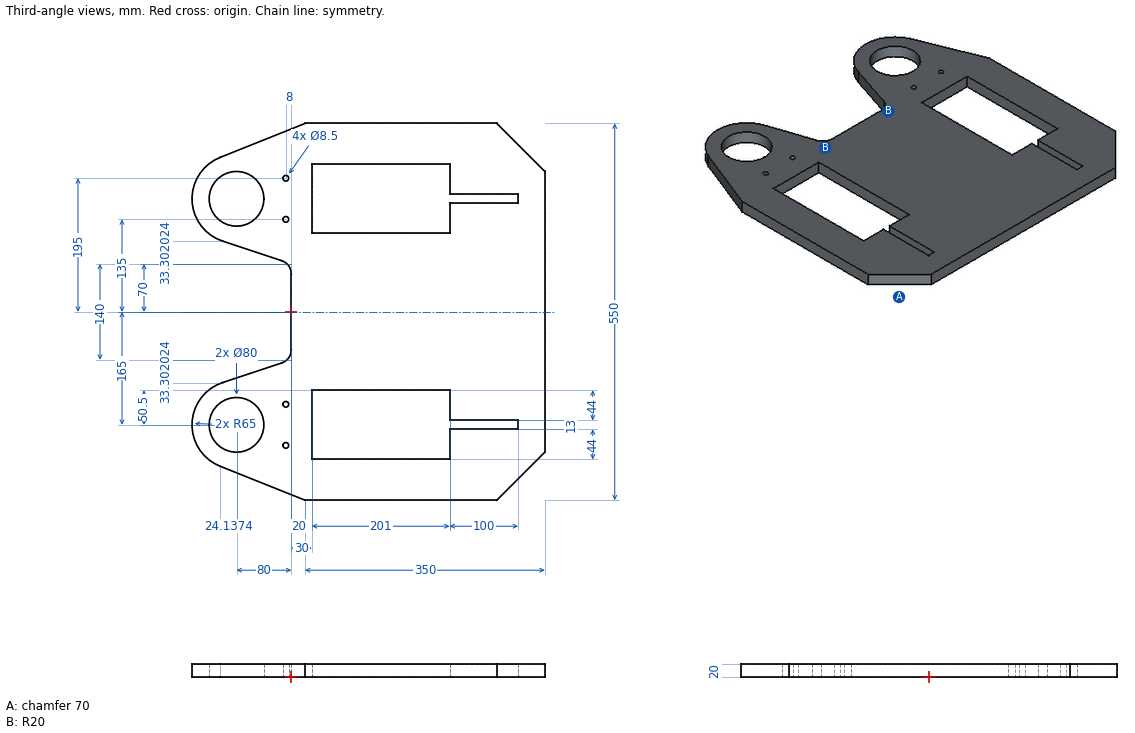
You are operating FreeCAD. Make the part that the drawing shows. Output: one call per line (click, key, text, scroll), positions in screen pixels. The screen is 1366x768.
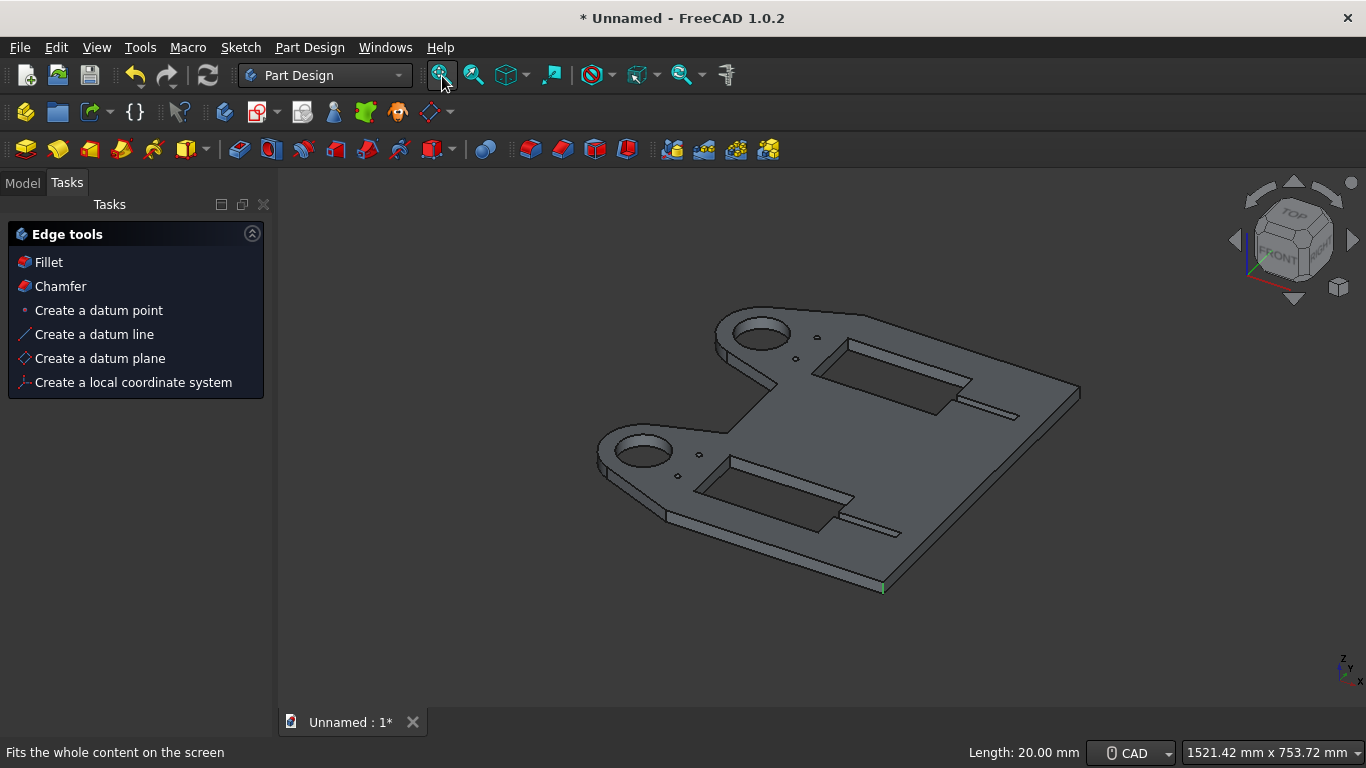
key(0)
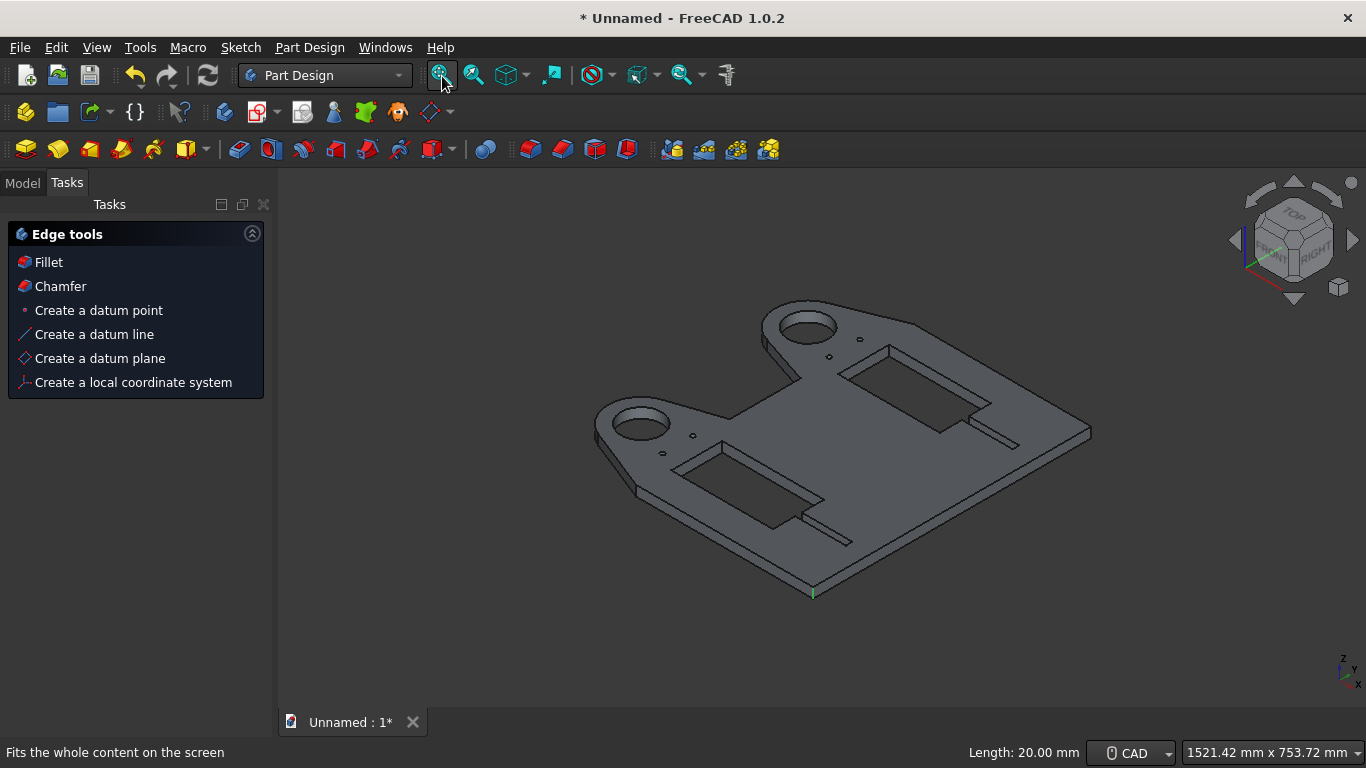
scroll(1091, 431, up, 6)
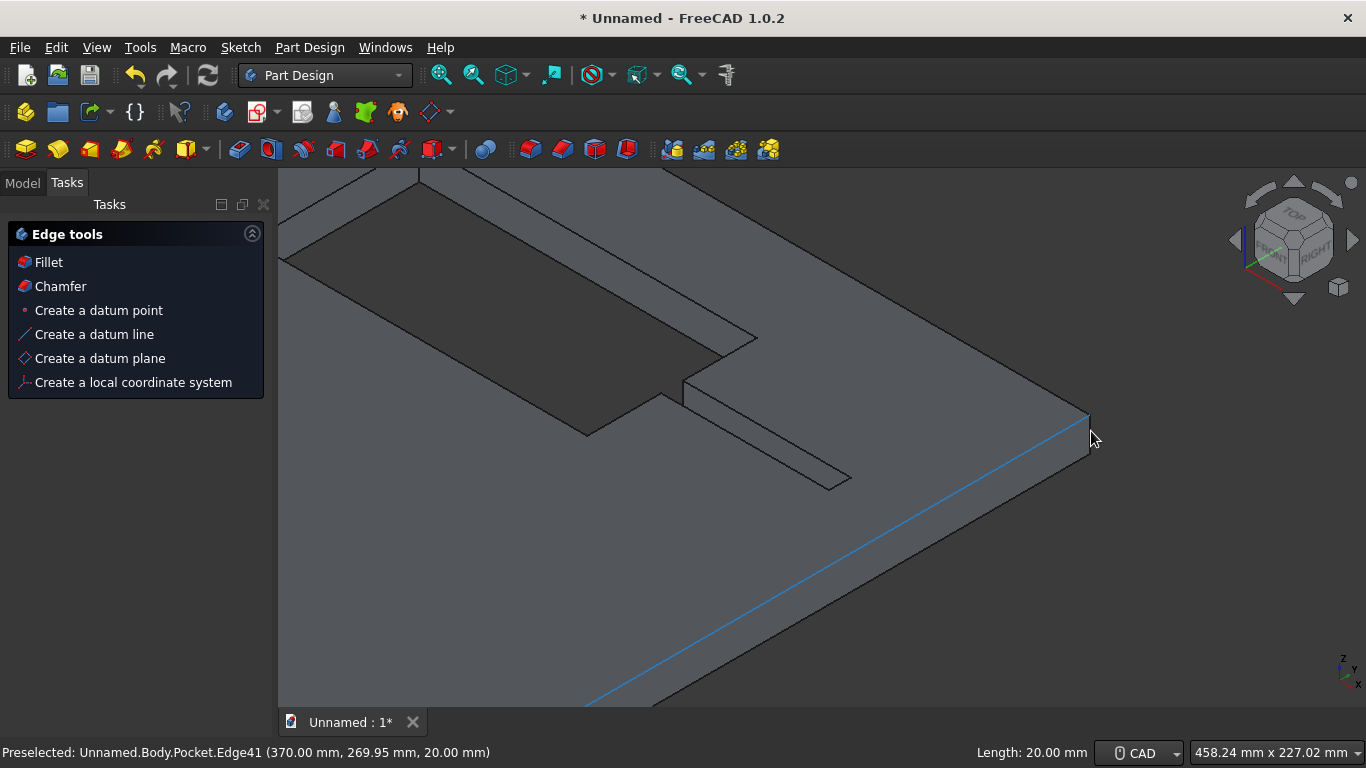
click(442, 76)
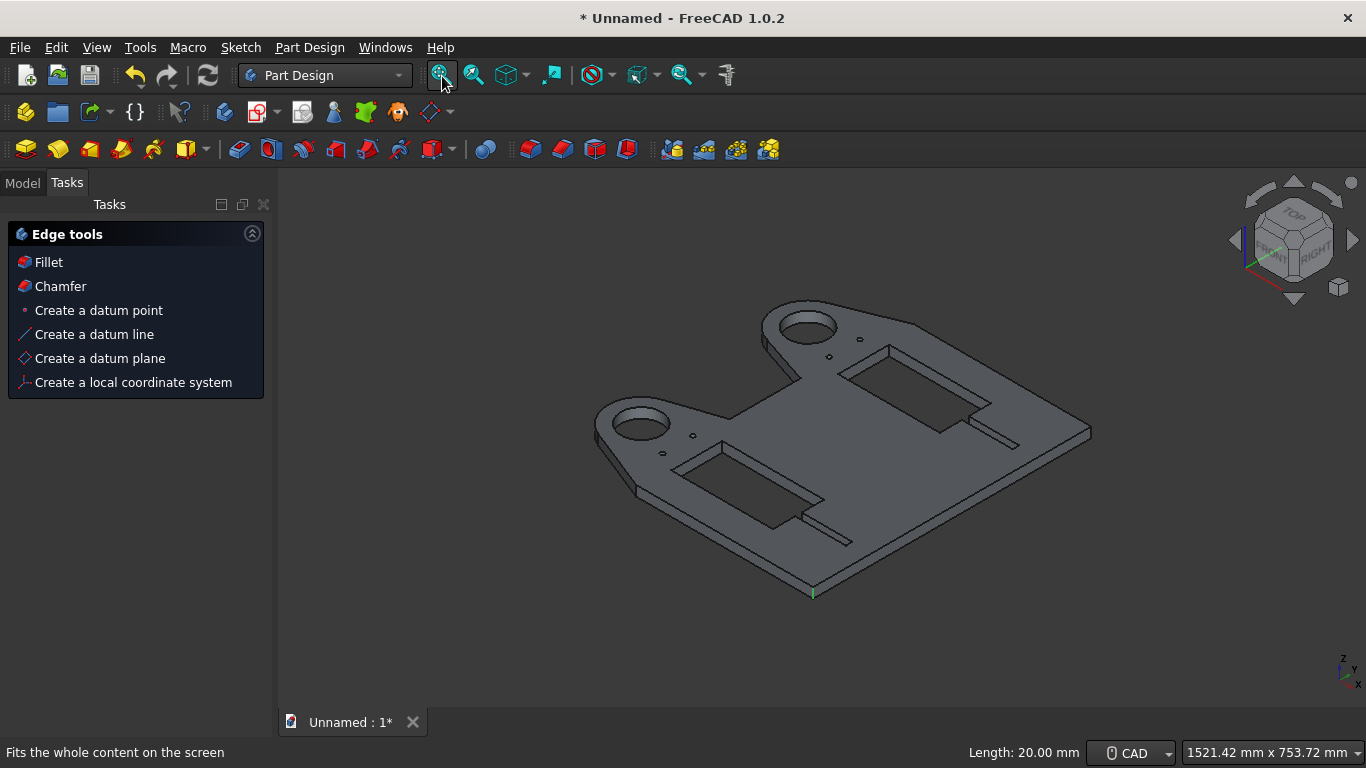
key(2)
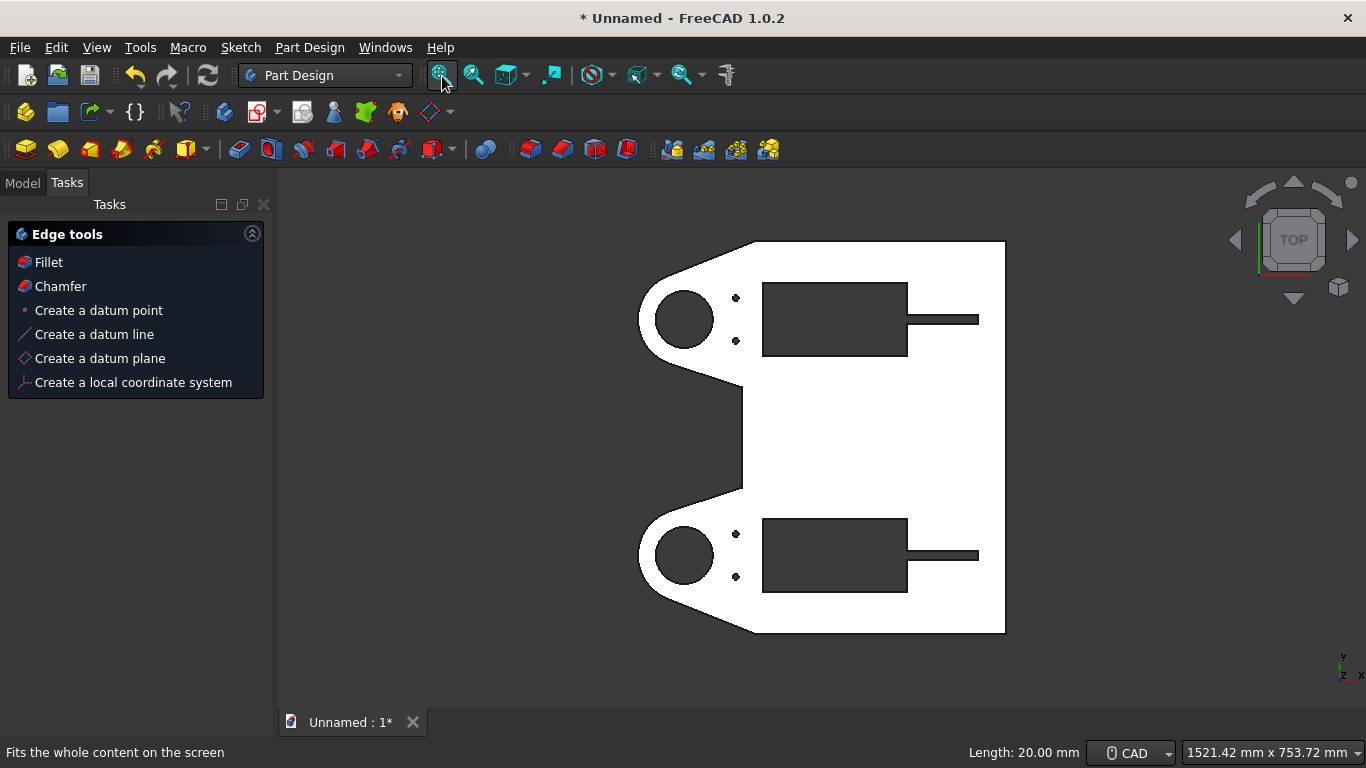
scroll(1006, 240, up, 6)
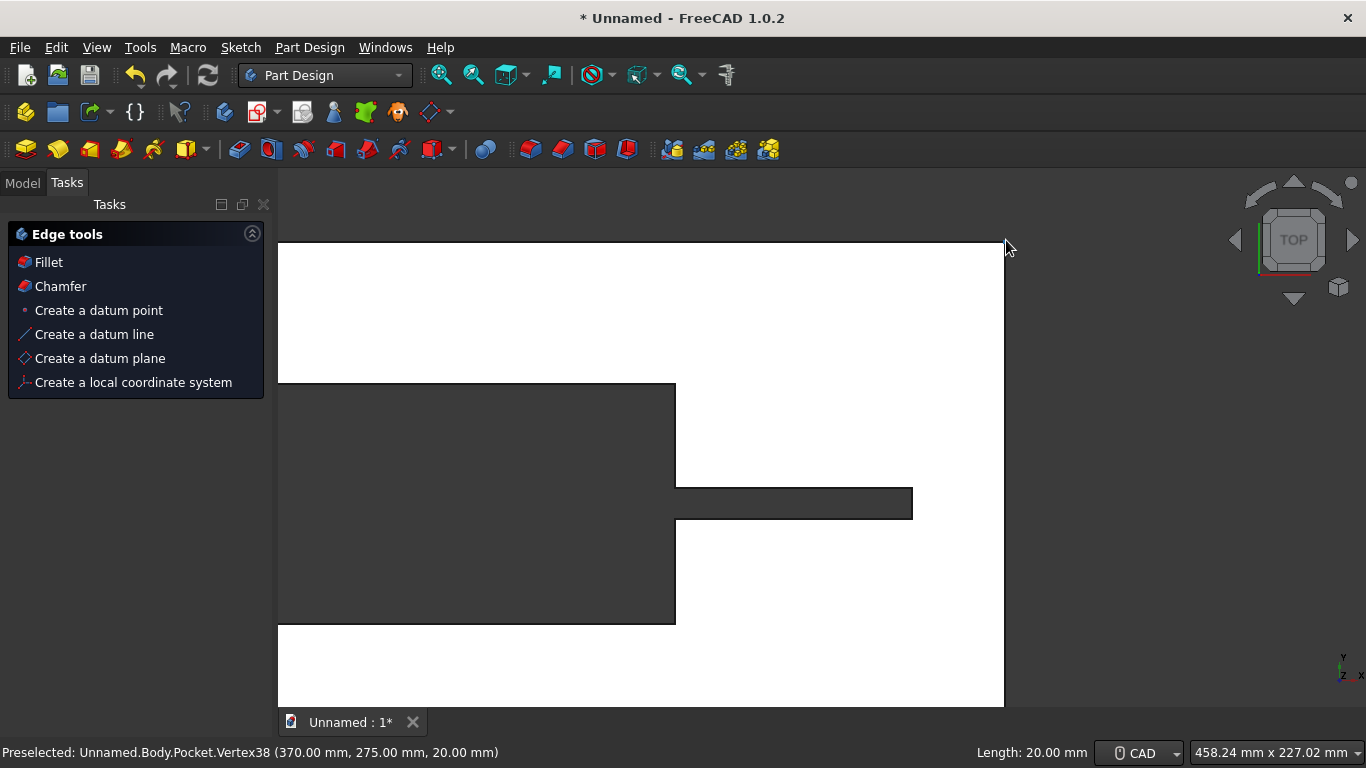
key(v)
key(f)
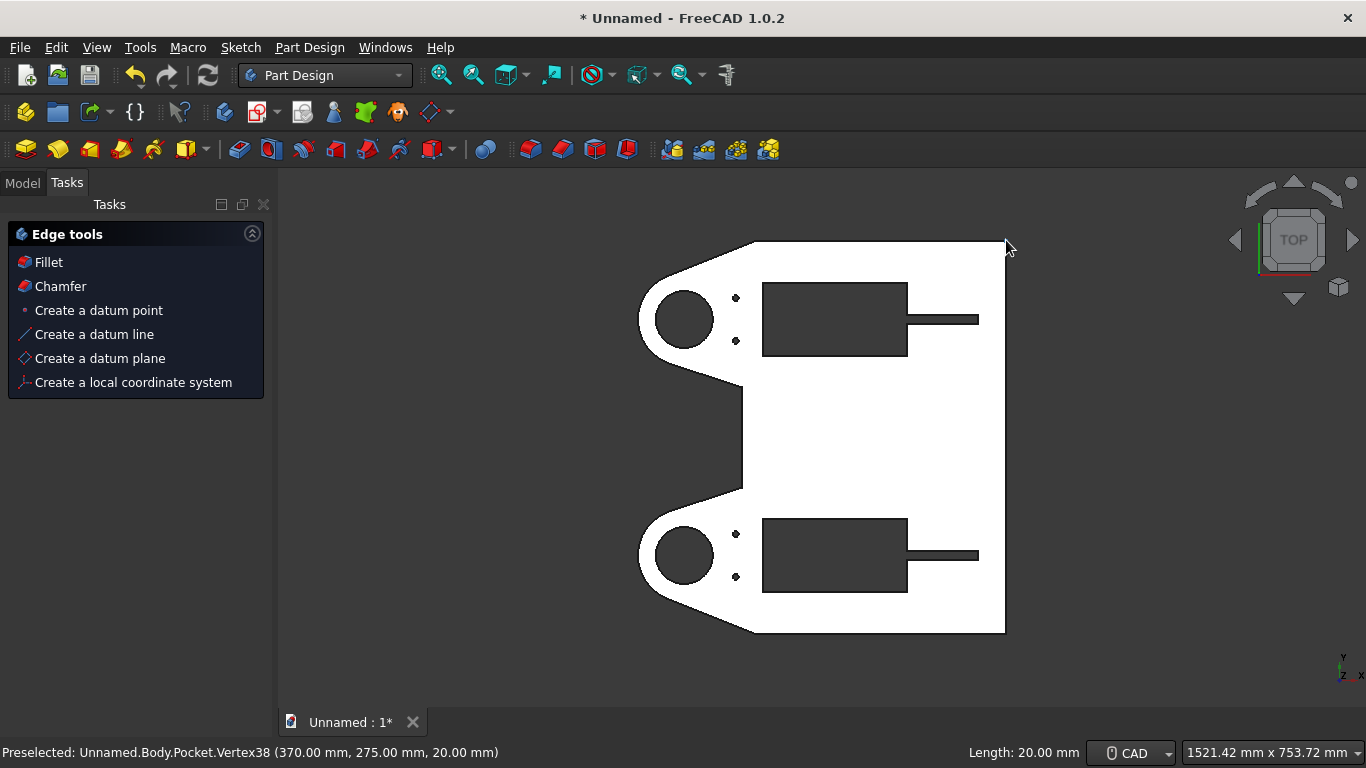
key(1)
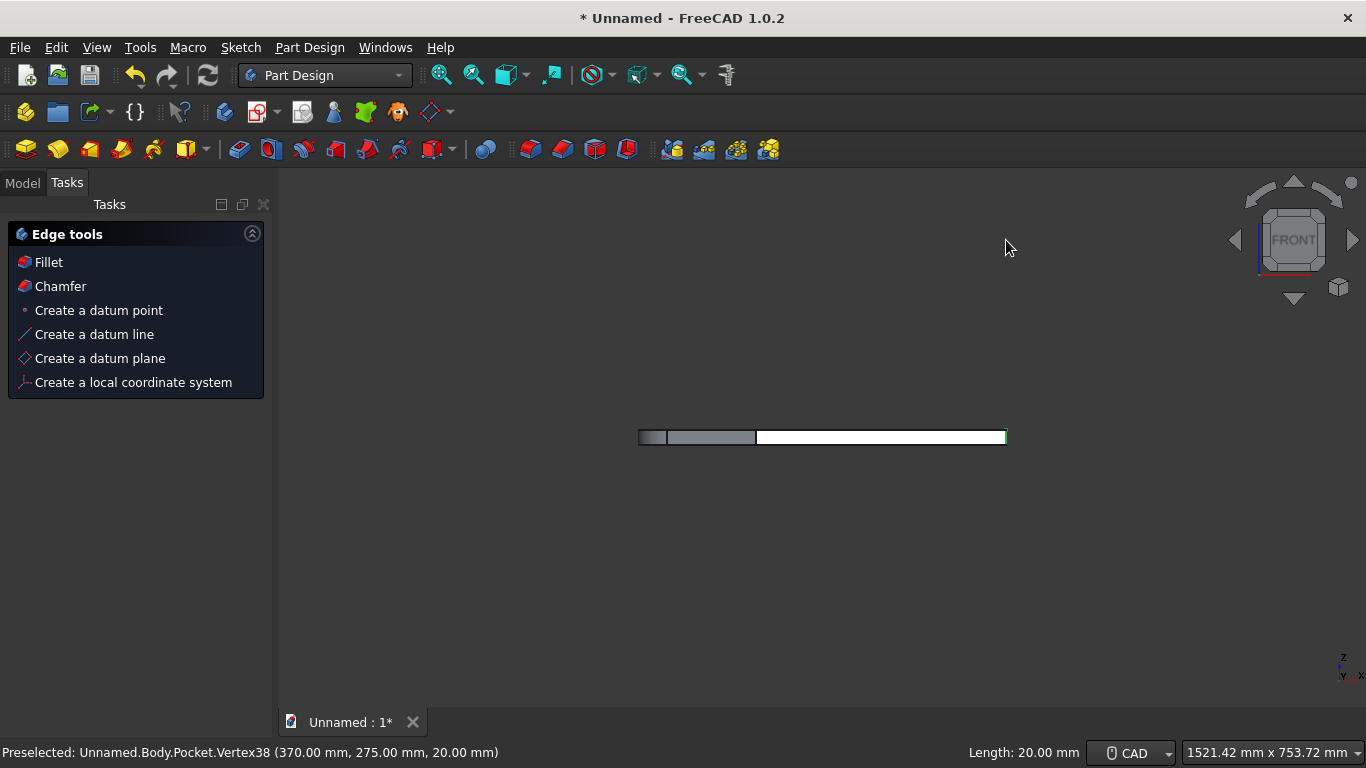
click(442, 76)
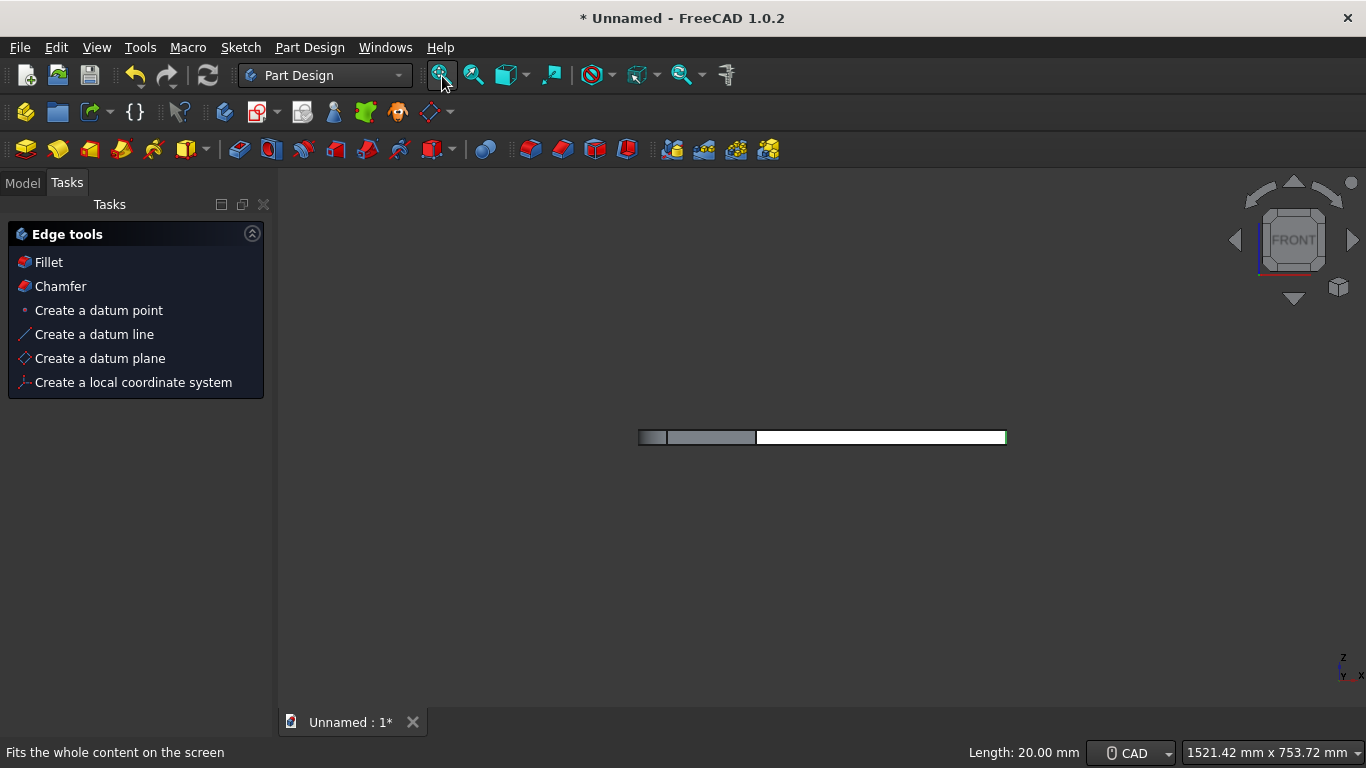
scroll(1006, 437, up, 6)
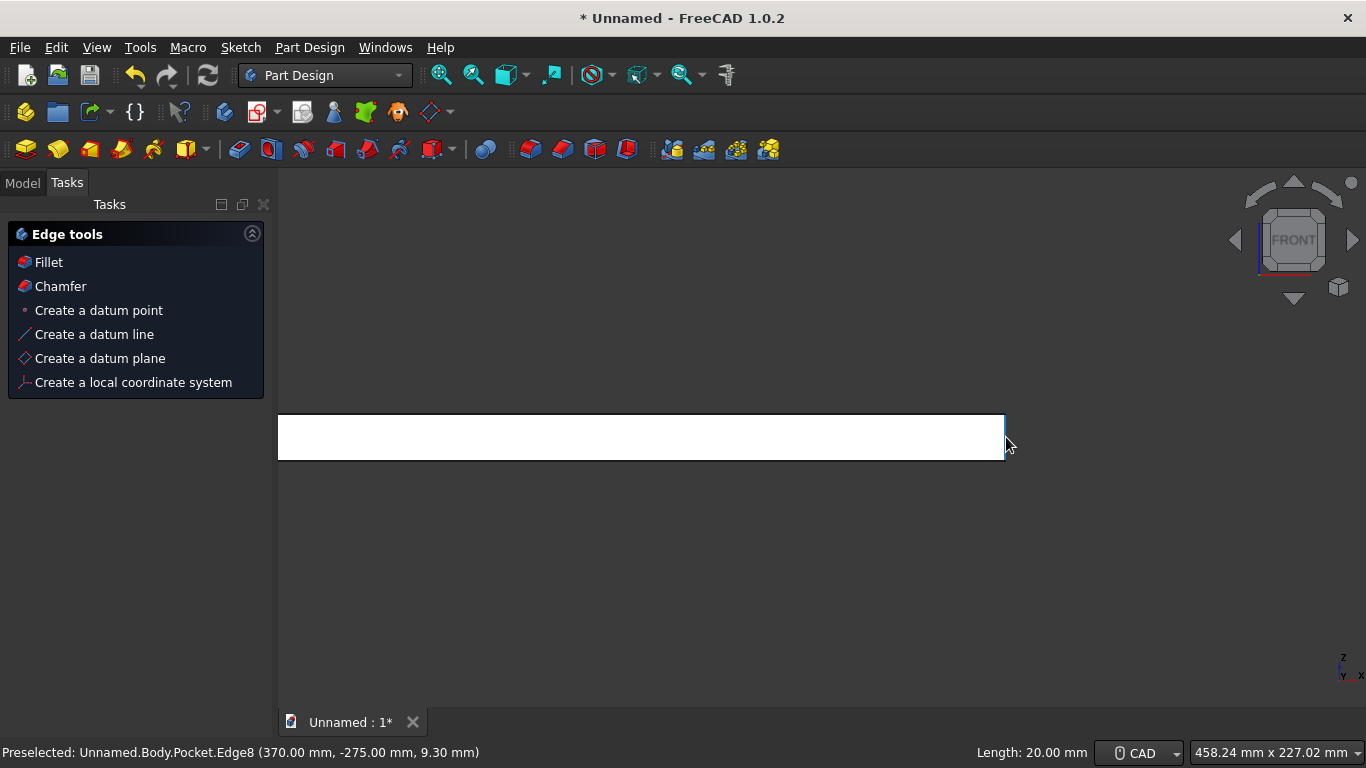
key(v)
key(f)